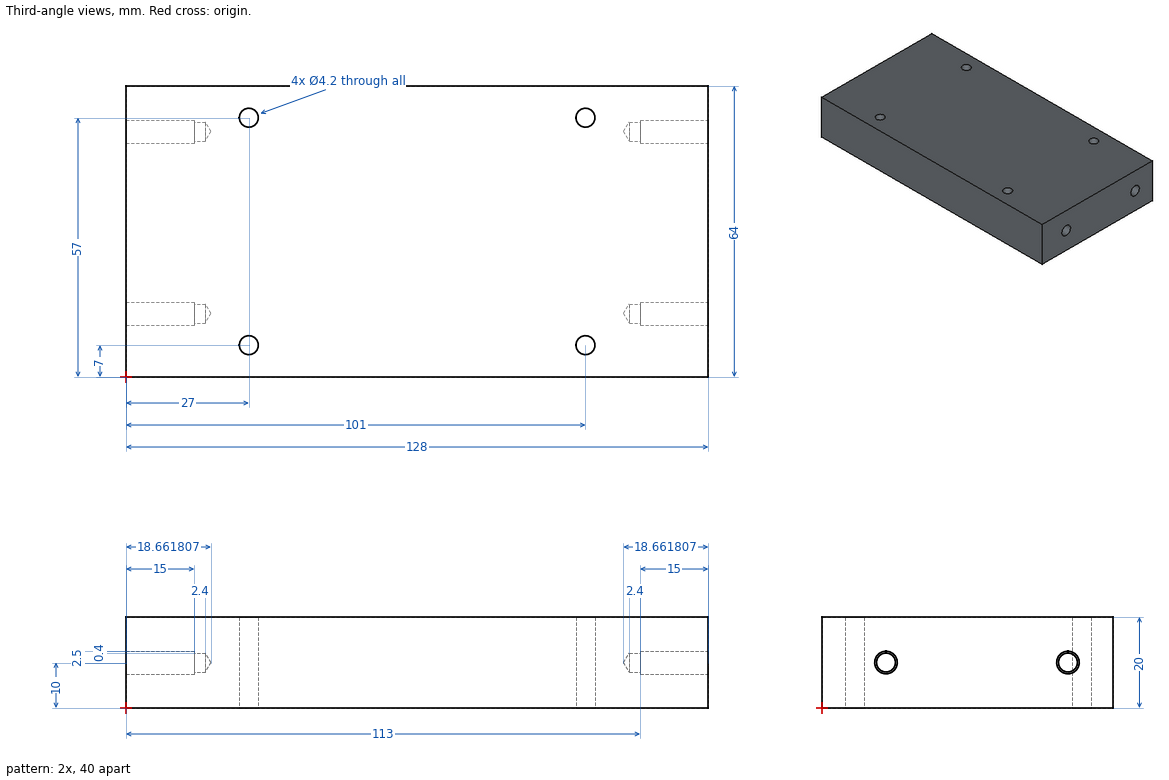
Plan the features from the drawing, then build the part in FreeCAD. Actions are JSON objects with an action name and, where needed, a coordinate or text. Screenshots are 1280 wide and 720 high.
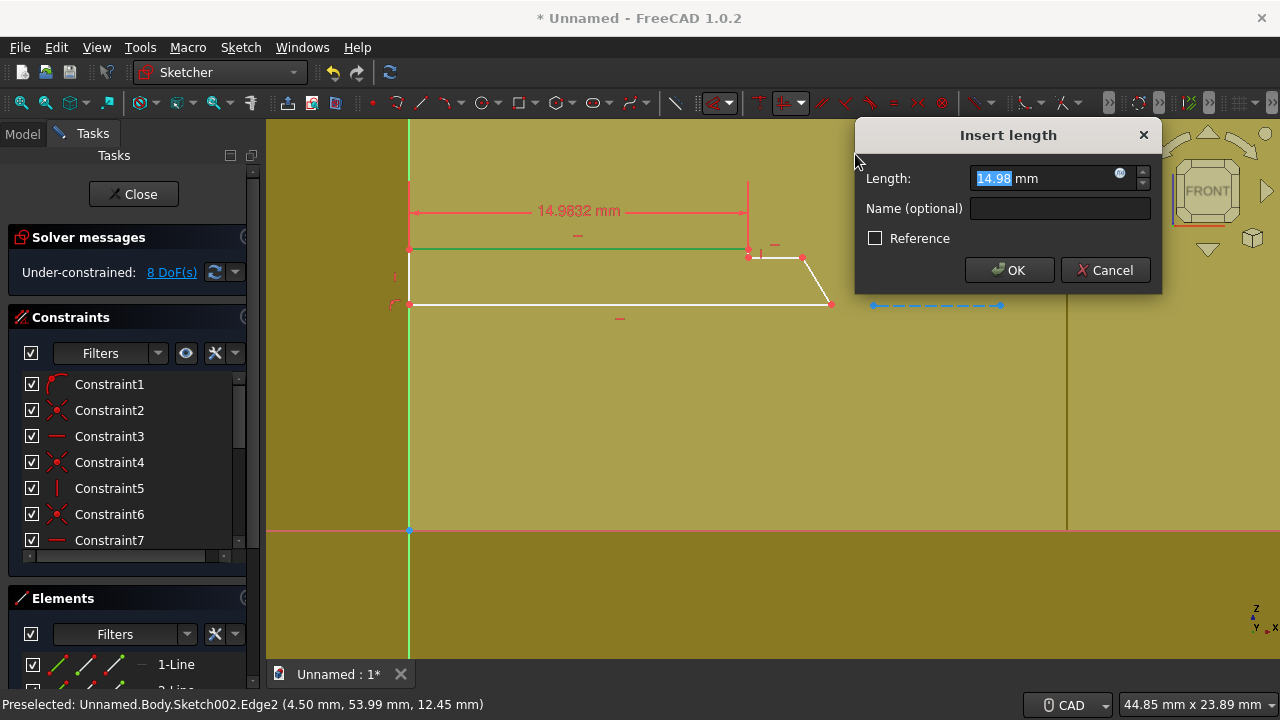
{"action": "type", "text": "15"}
{"action": "key", "text": "Return"}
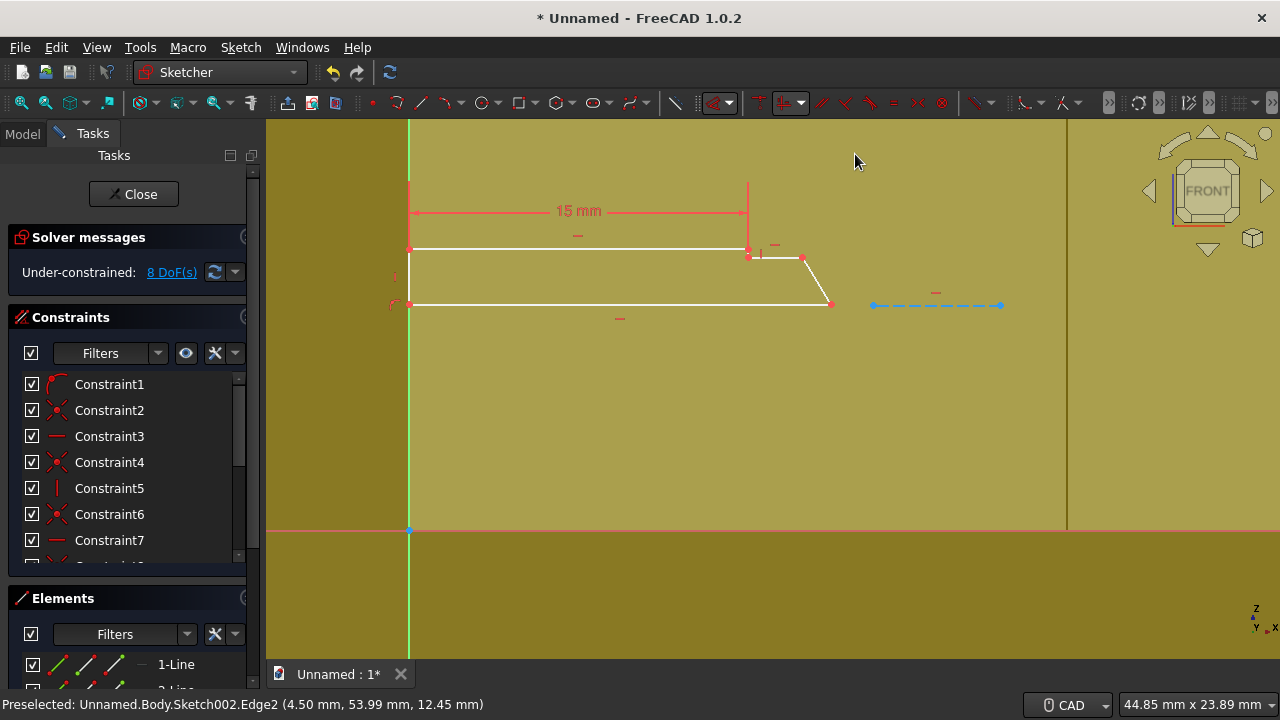
{"action": "left_click", "coordinate": [409, 288]}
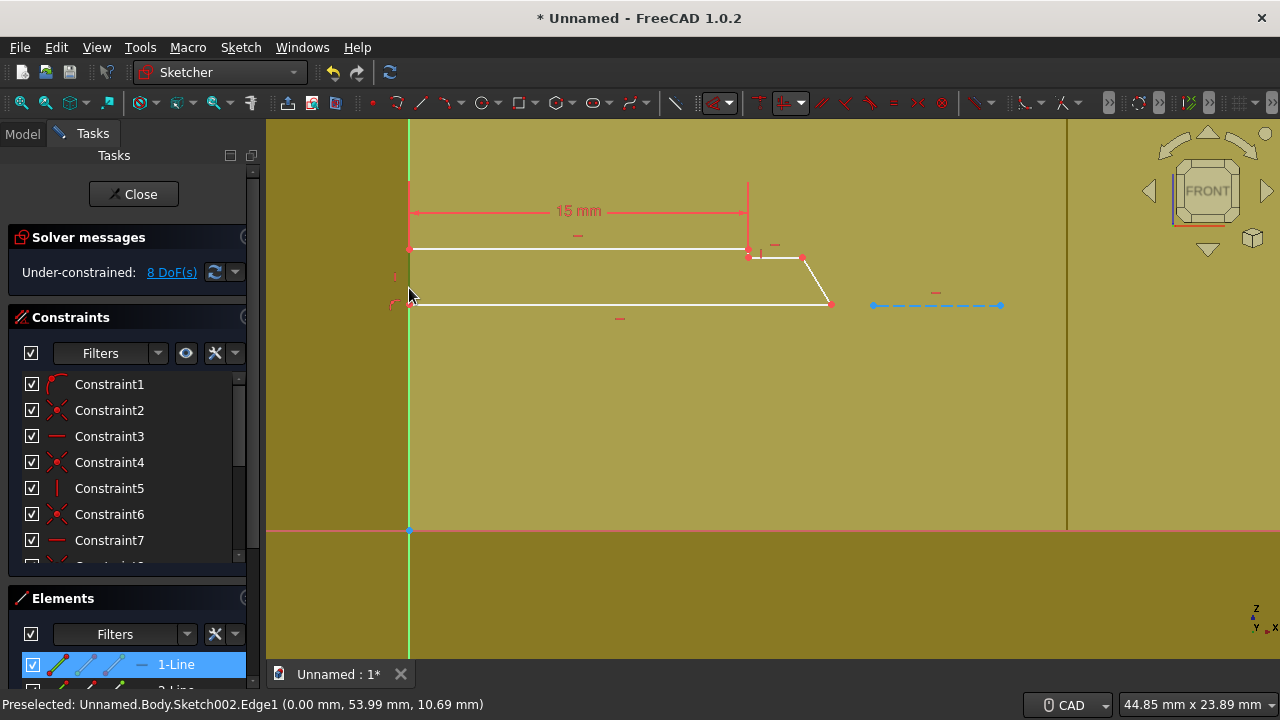
{"action": "left_click", "coordinate": [732, 104]}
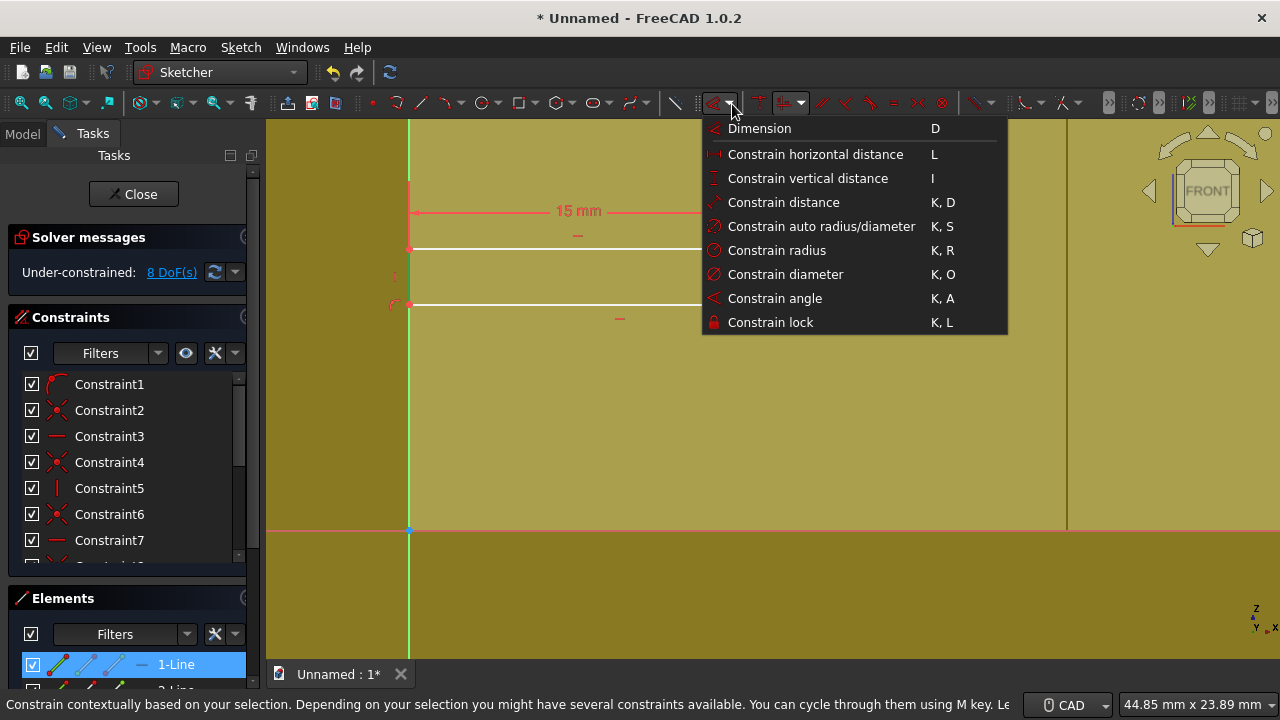
{"action": "left_click", "coordinate": [855, 178]}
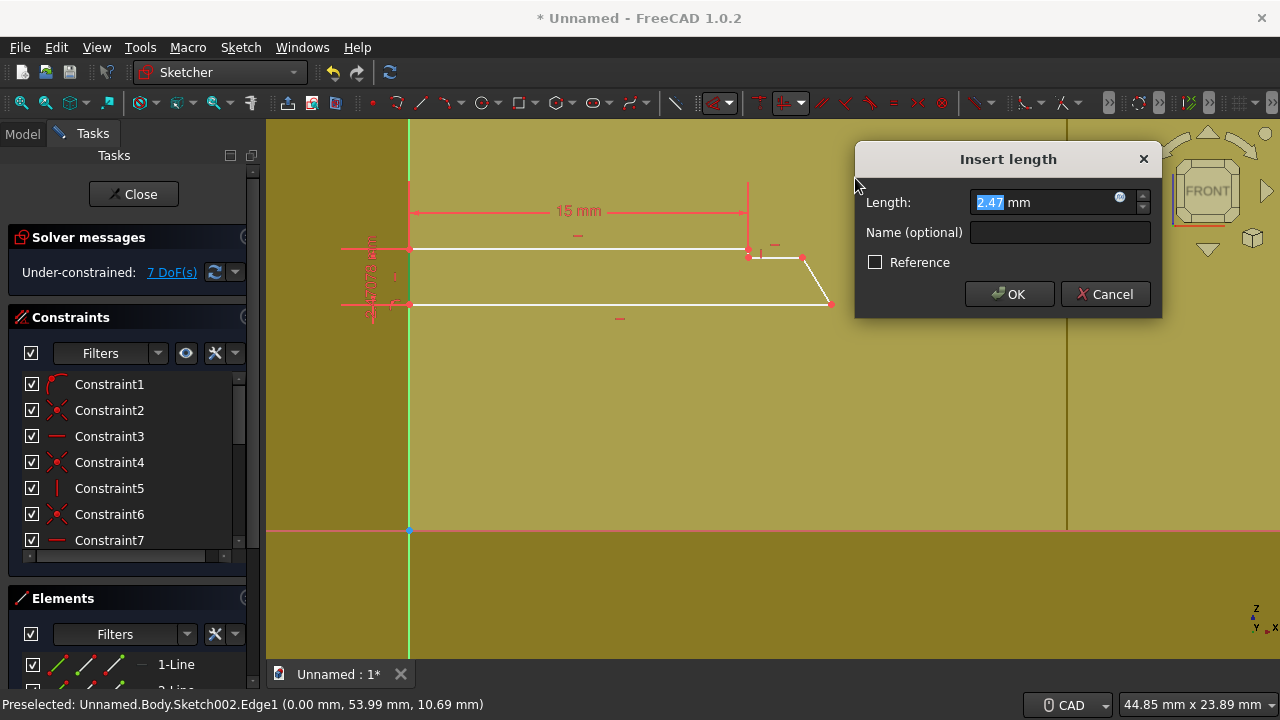
{"action": "type", "text": "2.5"}
{"action": "key", "text": "Return"}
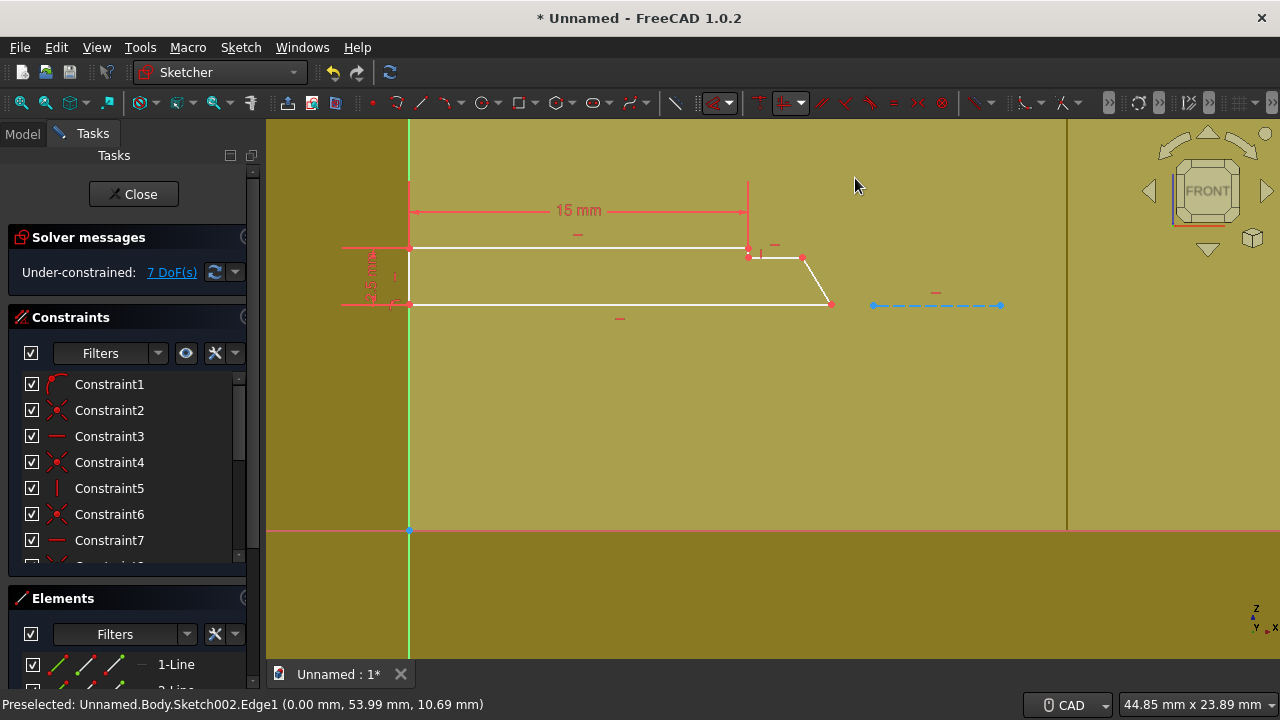
{"action": "scroll", "coordinate": [748, 253], "scroll_direction": "up", "scroll_amount": 8}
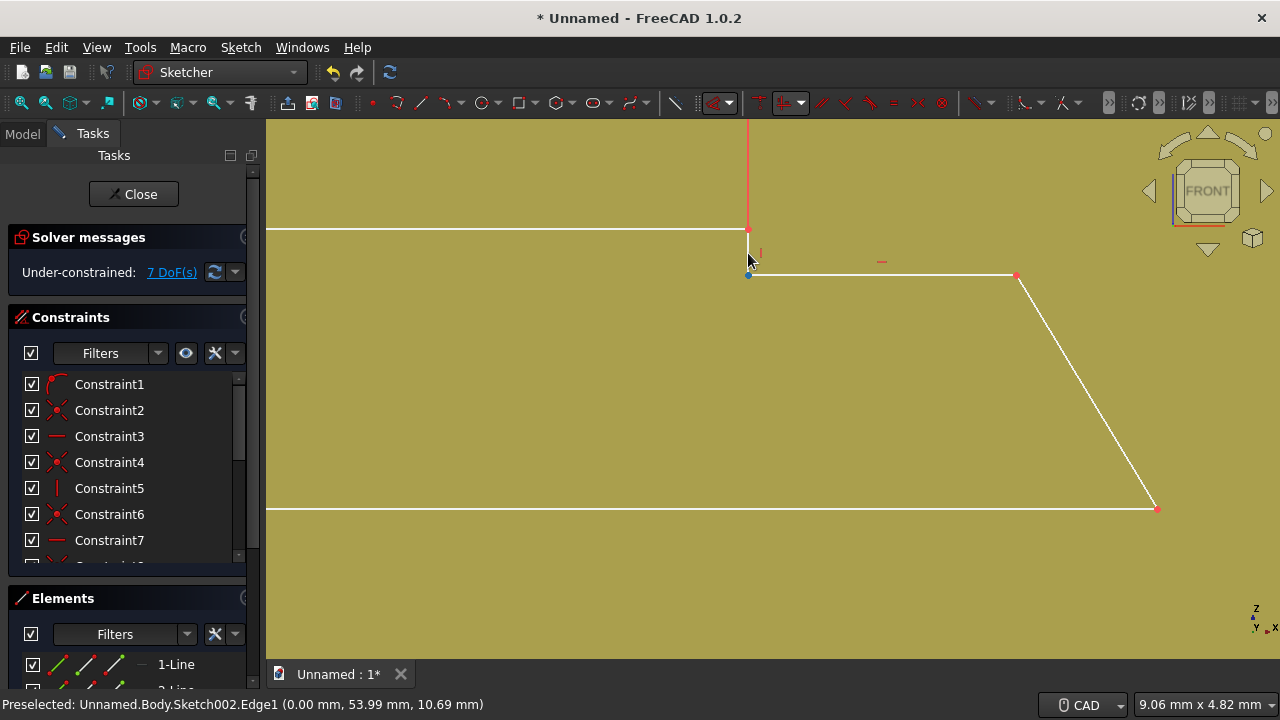
{"action": "left_click", "coordinate": [748, 252]}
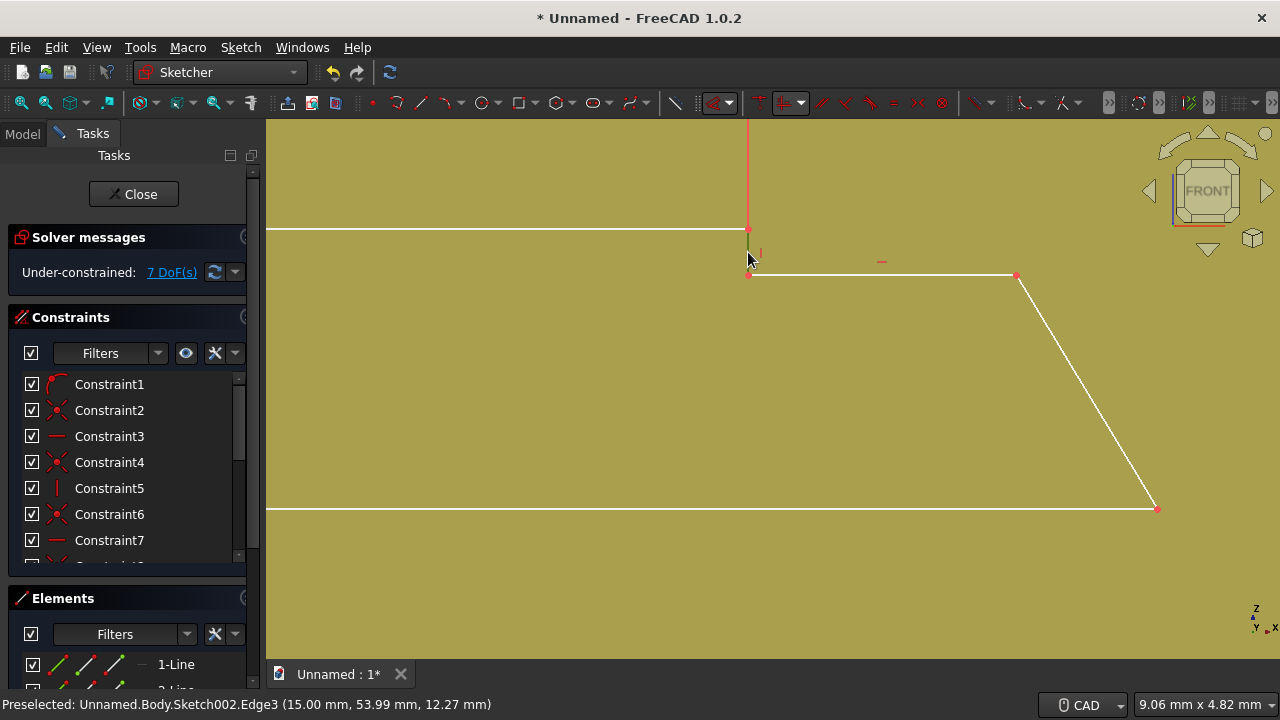
{"action": "key", "text": "i"}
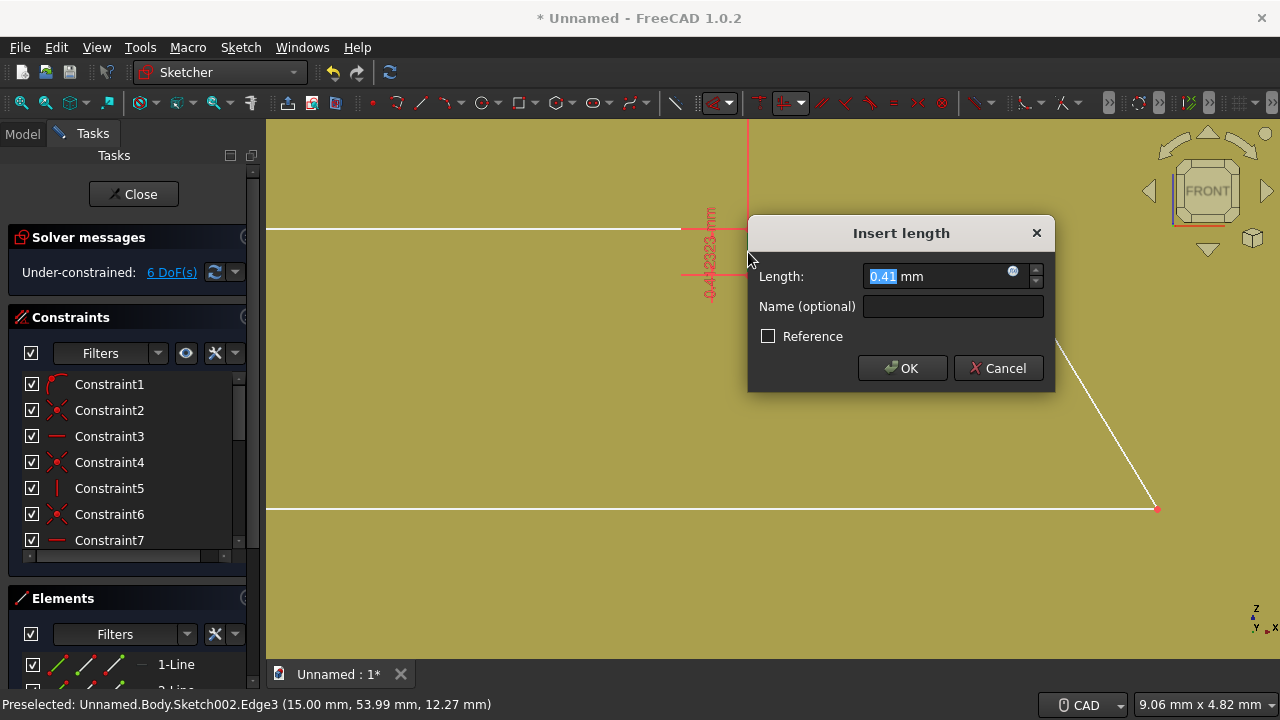
{"action": "type", "text": "0.4"}
{"action": "key", "text": "Return"}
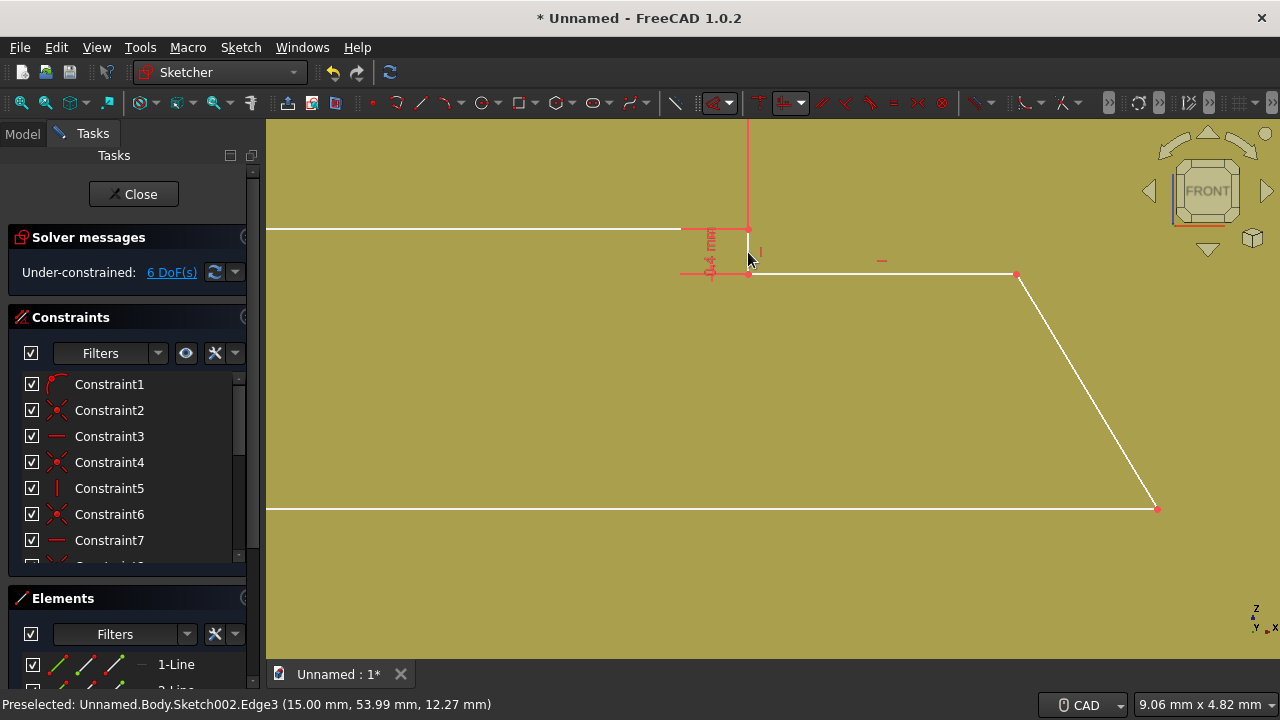
{"action": "scroll", "coordinate": [748, 253], "scroll_direction": "down", "scroll_amount": 8}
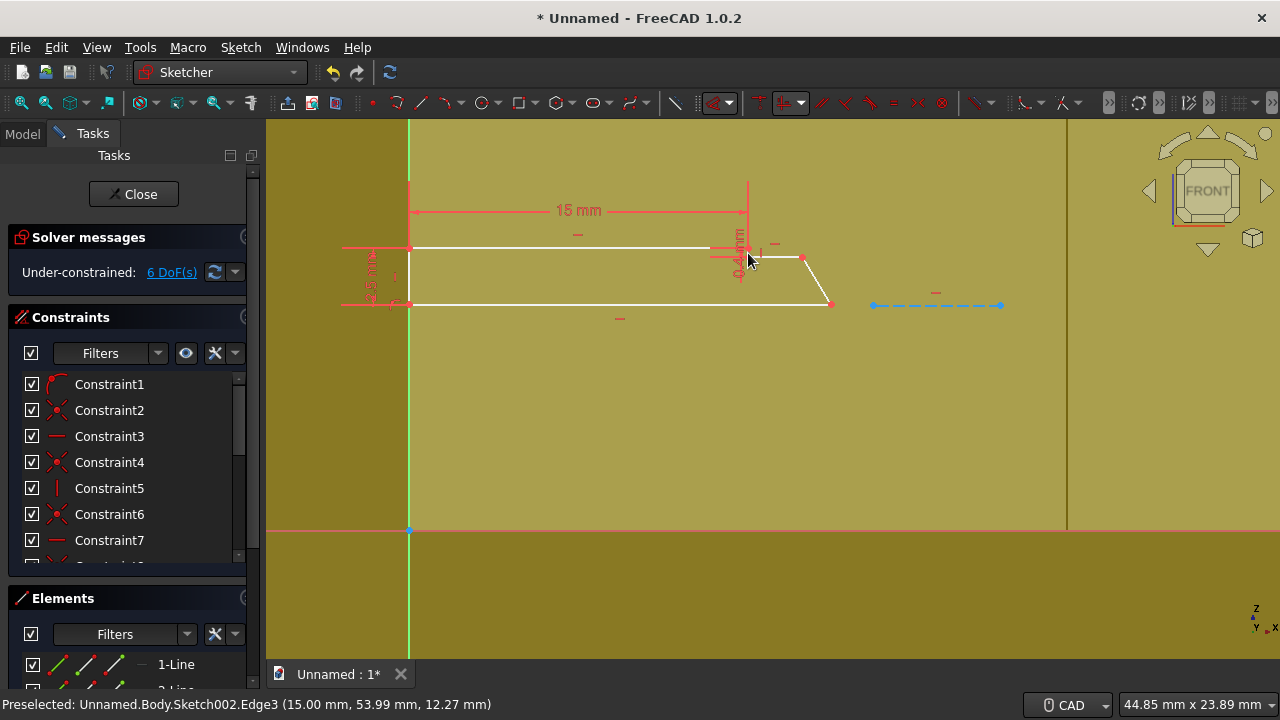
{"action": "left_click", "coordinate": [786, 257]}